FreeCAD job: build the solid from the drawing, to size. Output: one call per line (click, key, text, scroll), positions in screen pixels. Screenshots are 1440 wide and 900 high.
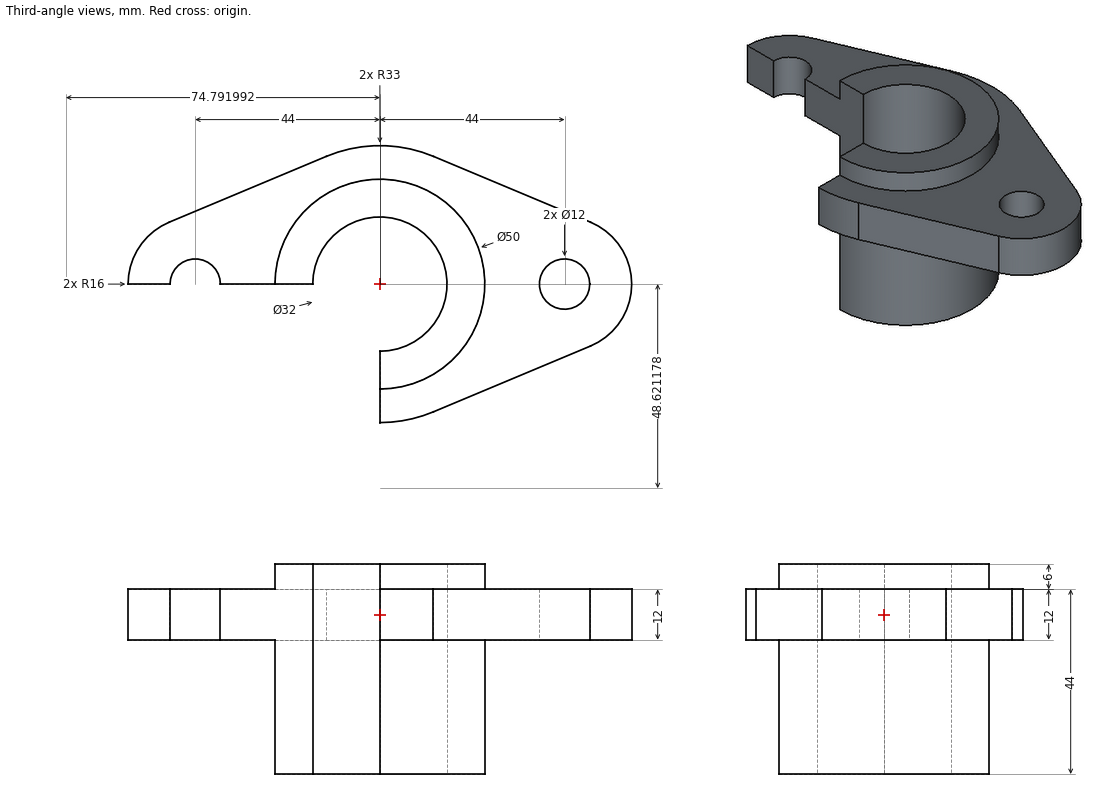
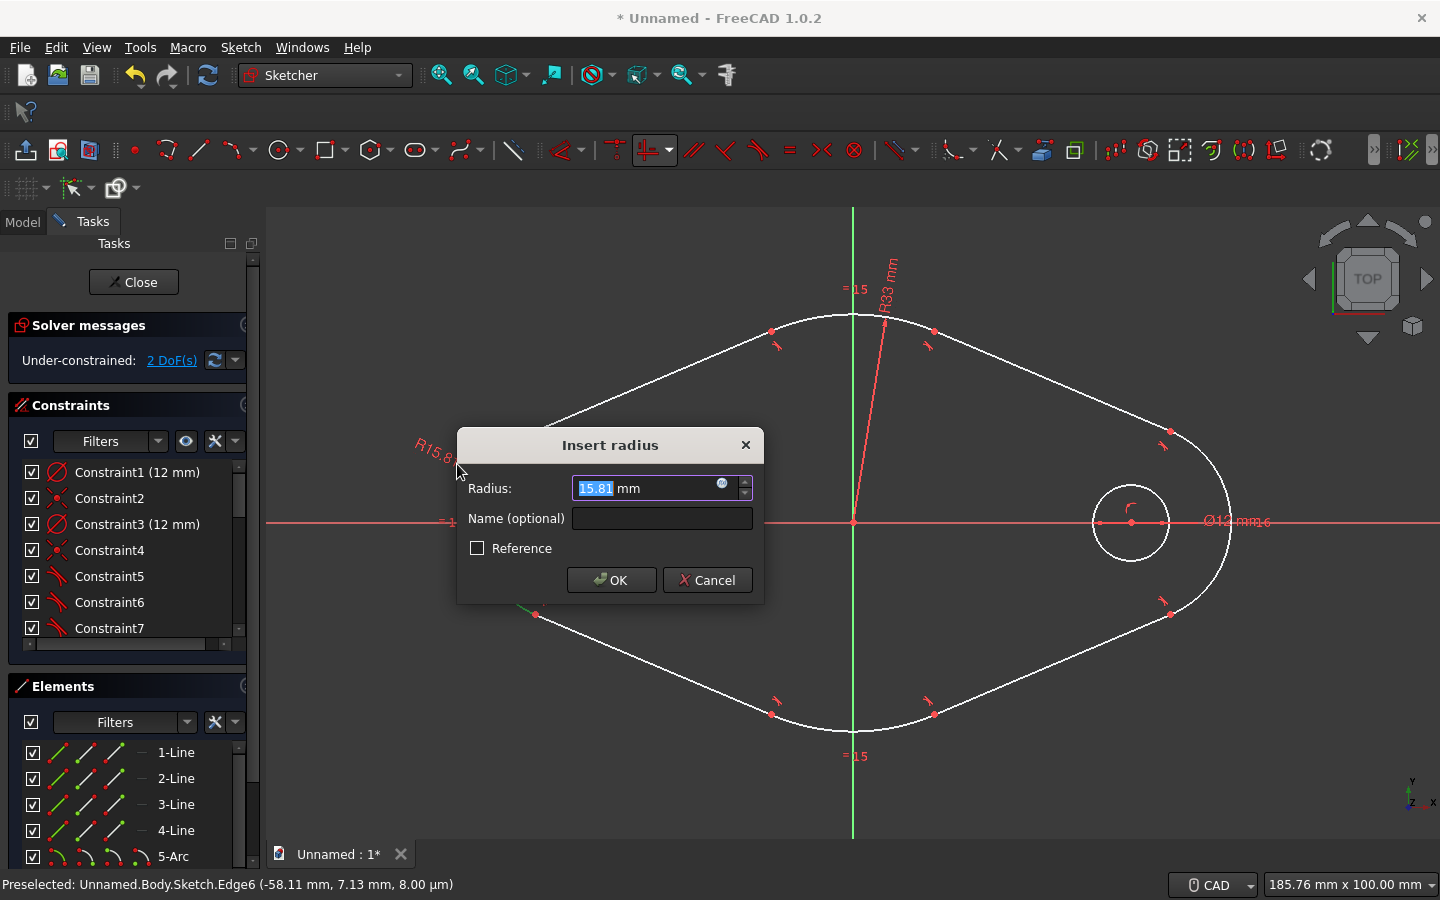
text(16)
key(Return)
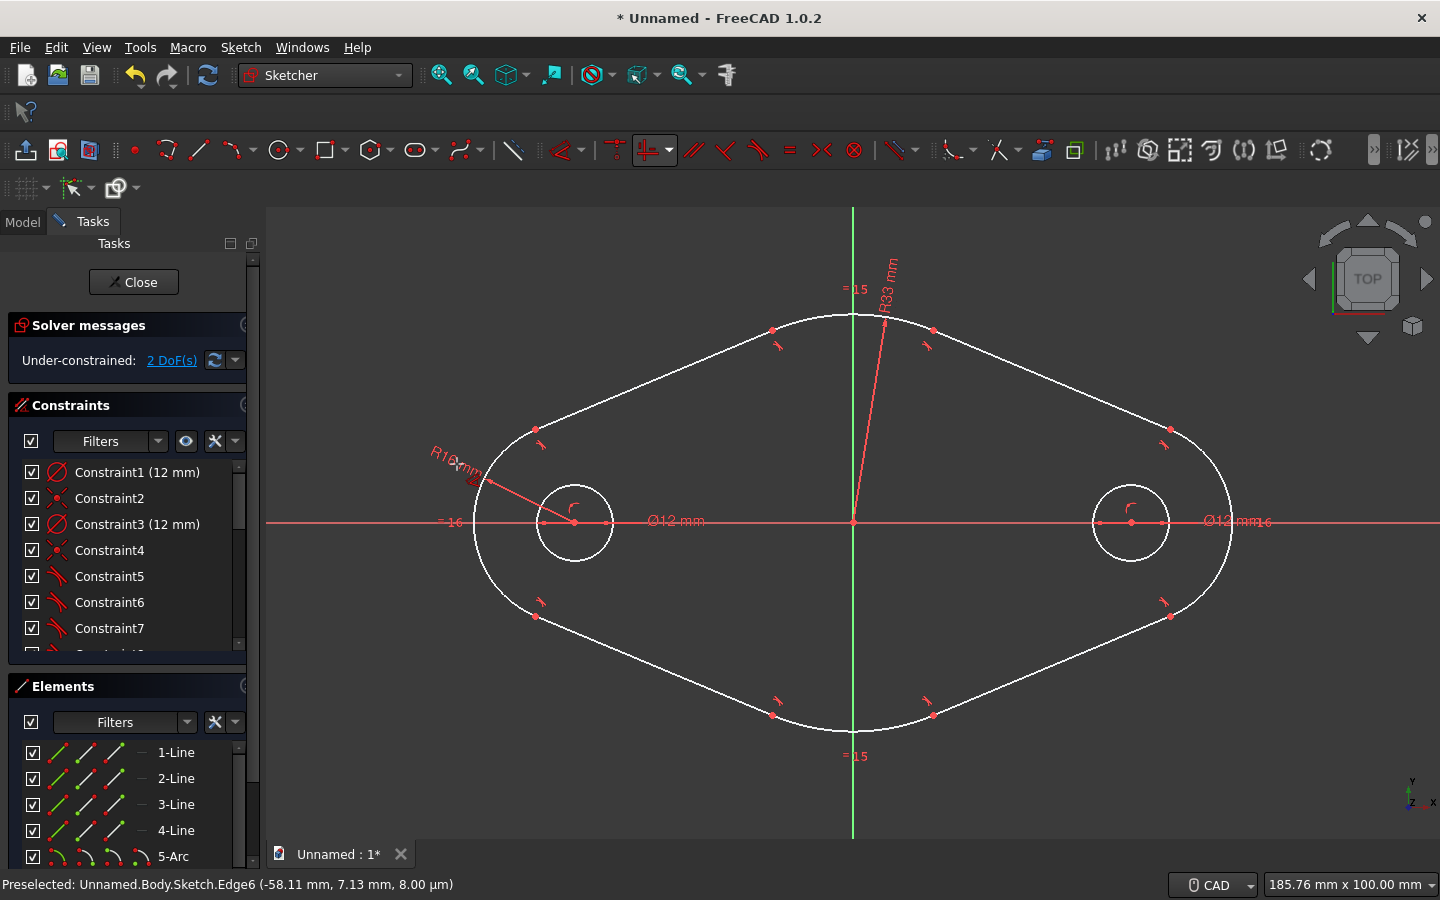
click(1131, 523)
click(992, 557)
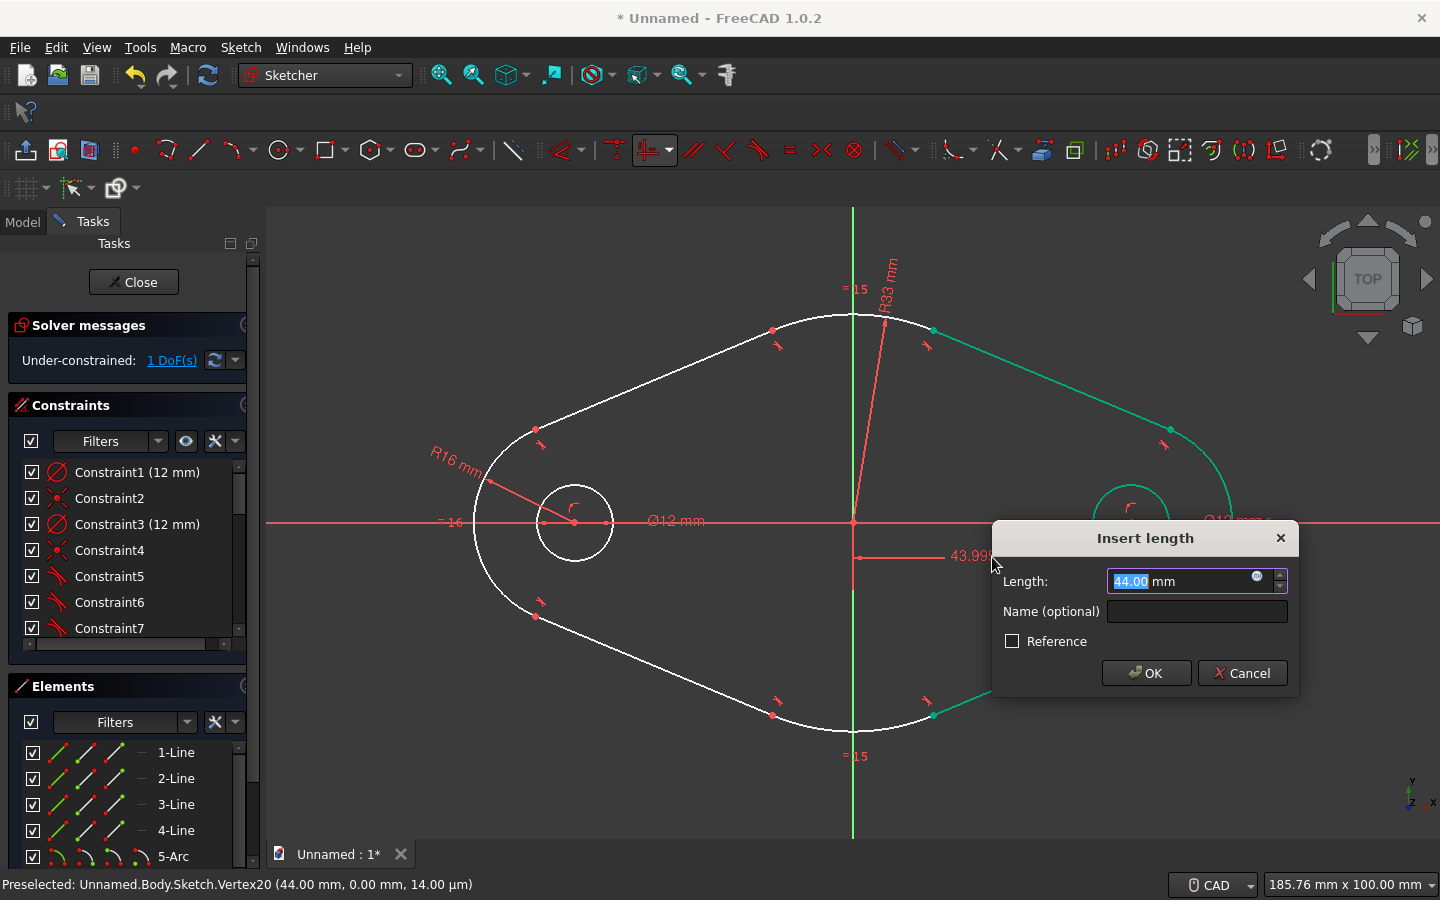
text(44)
key(Return)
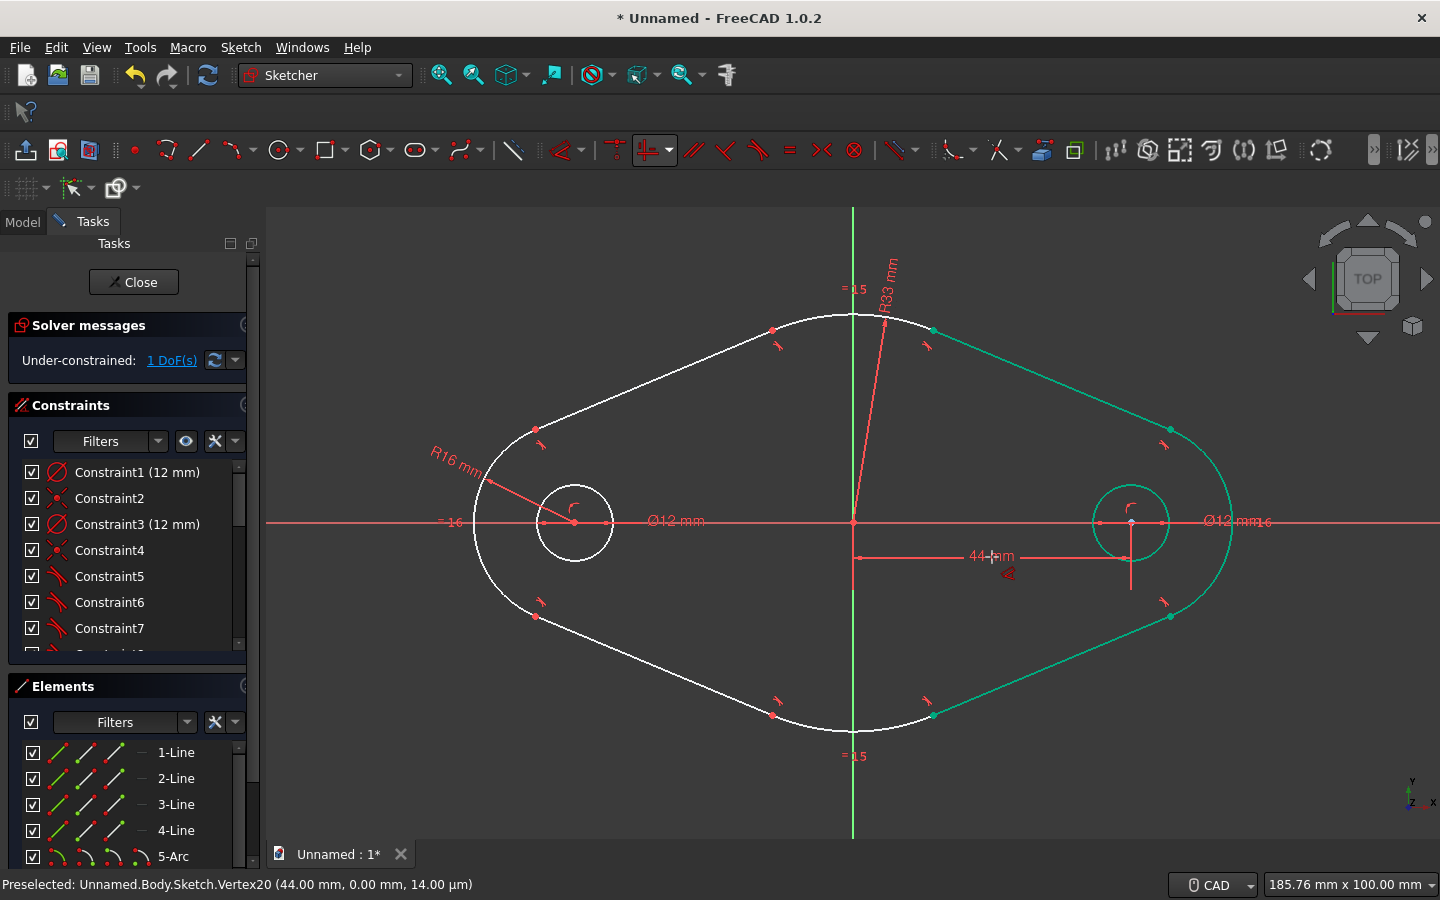
click(575, 523)
click(714, 557)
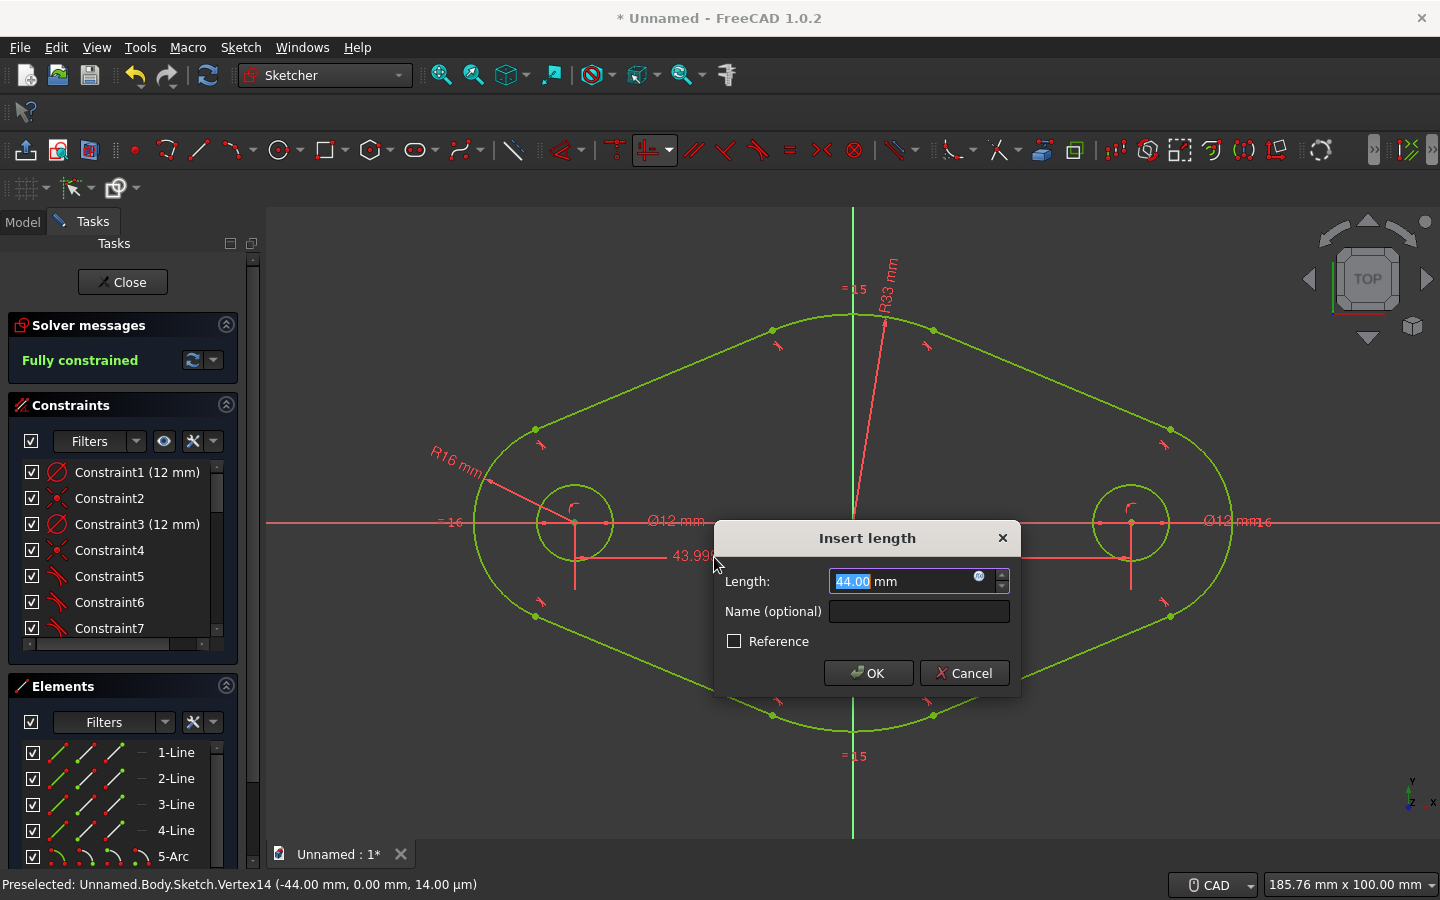
text(44)
key(Return)
key(Escape)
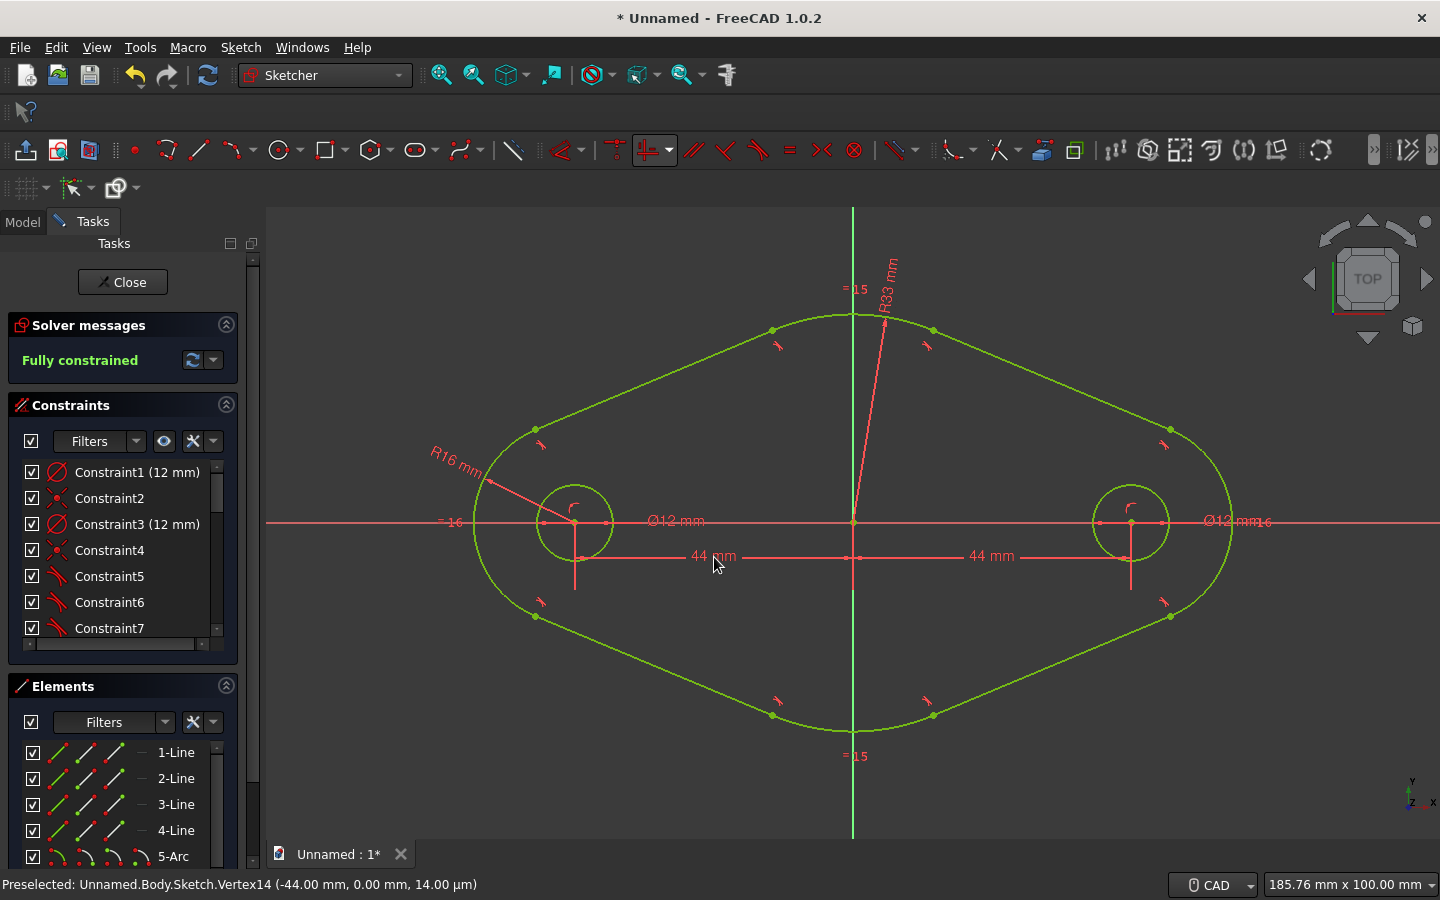
click(123, 282)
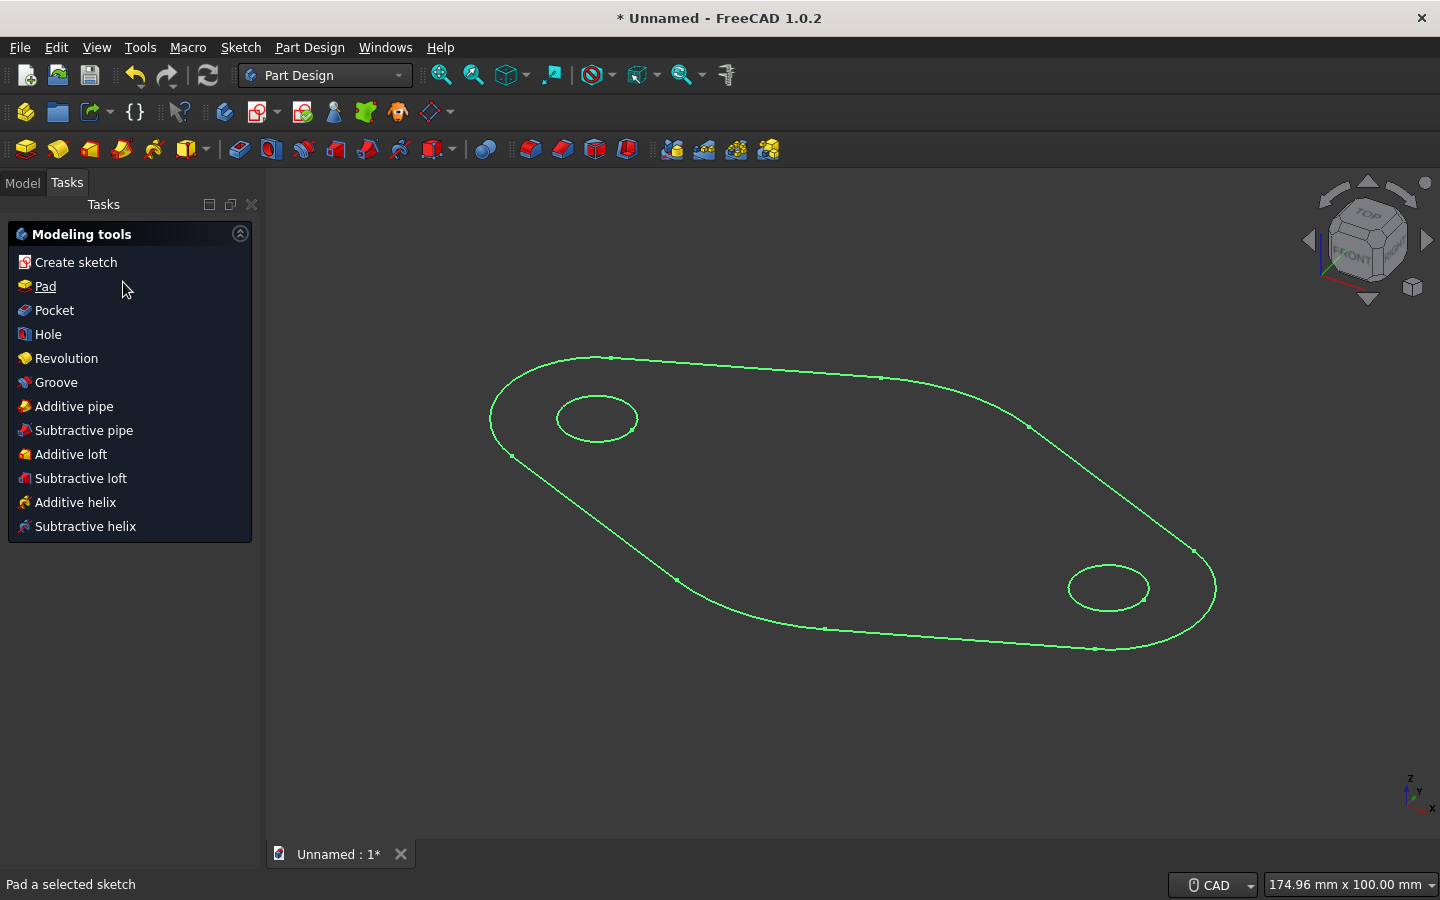
click(26, 150)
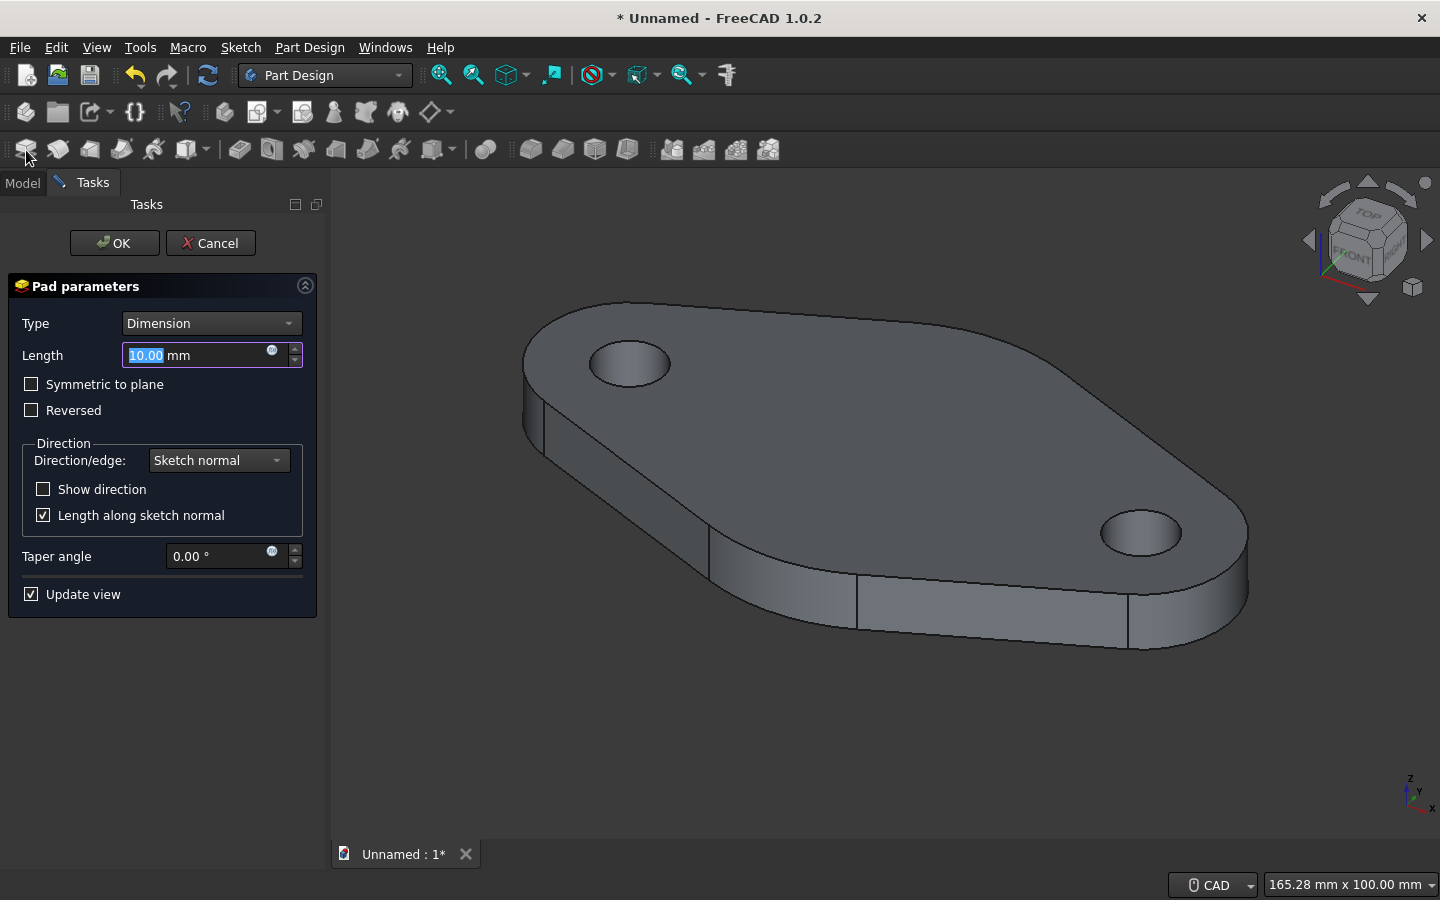
text(12)
key(Tab)